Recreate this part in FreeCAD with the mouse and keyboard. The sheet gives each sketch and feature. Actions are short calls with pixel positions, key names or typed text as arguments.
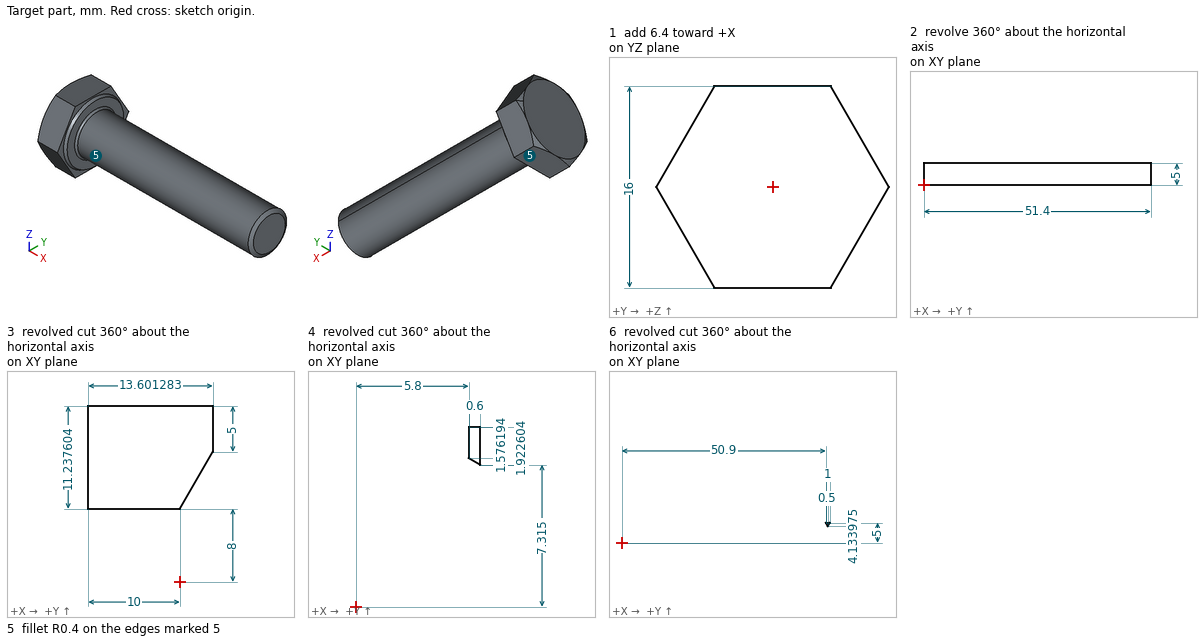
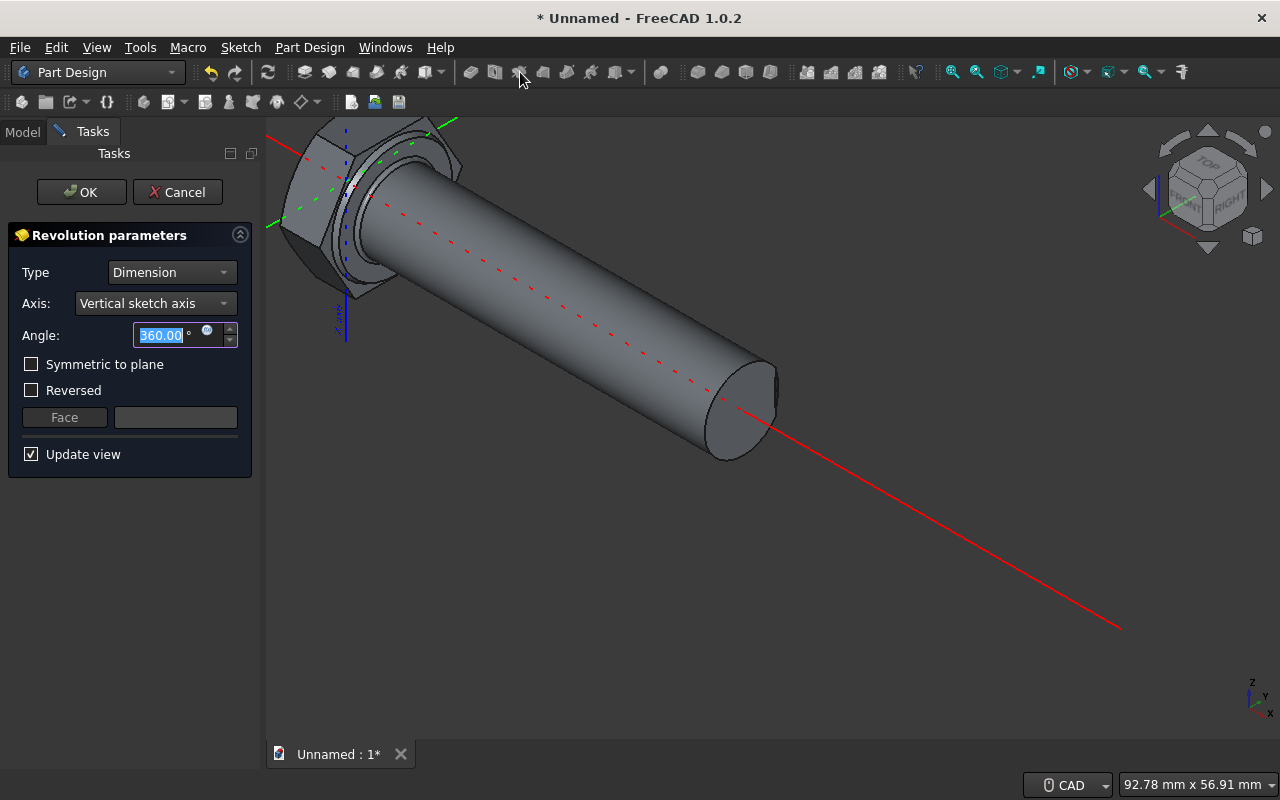
click(156, 304)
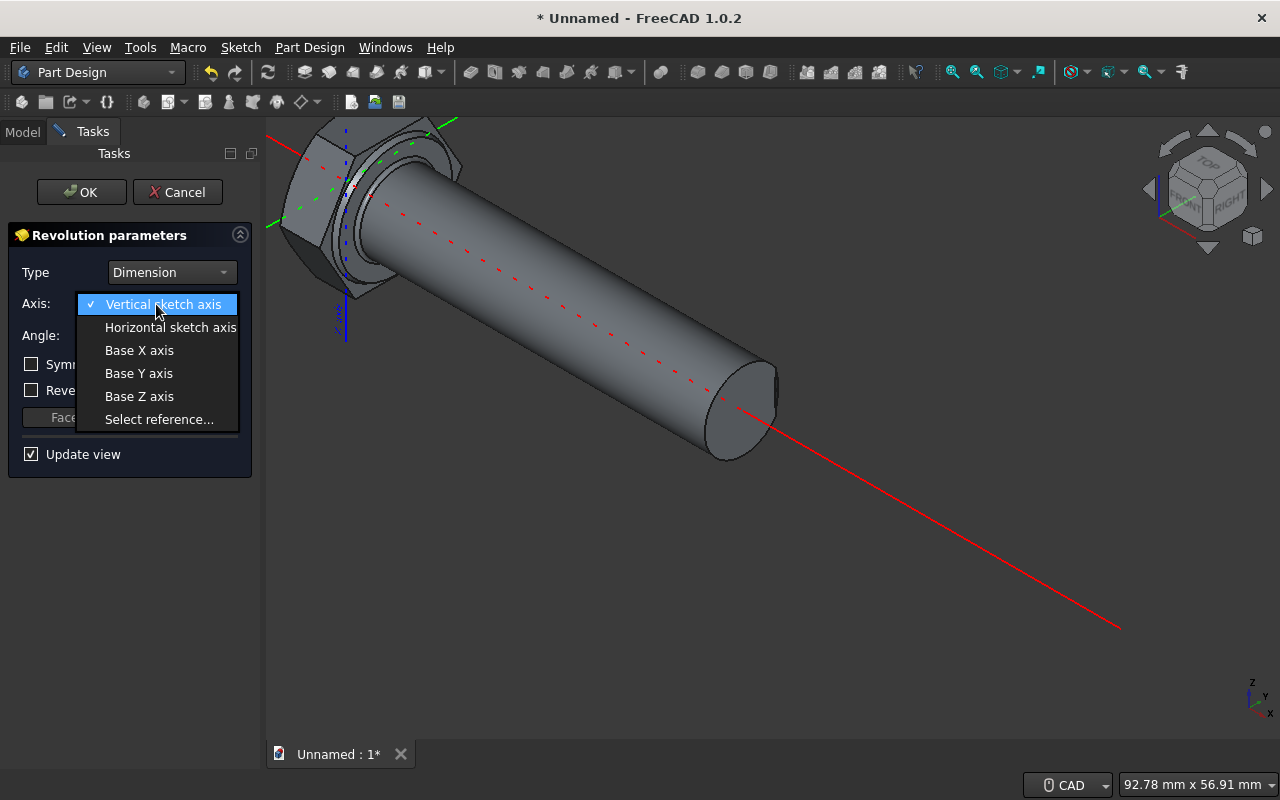
click(156, 328)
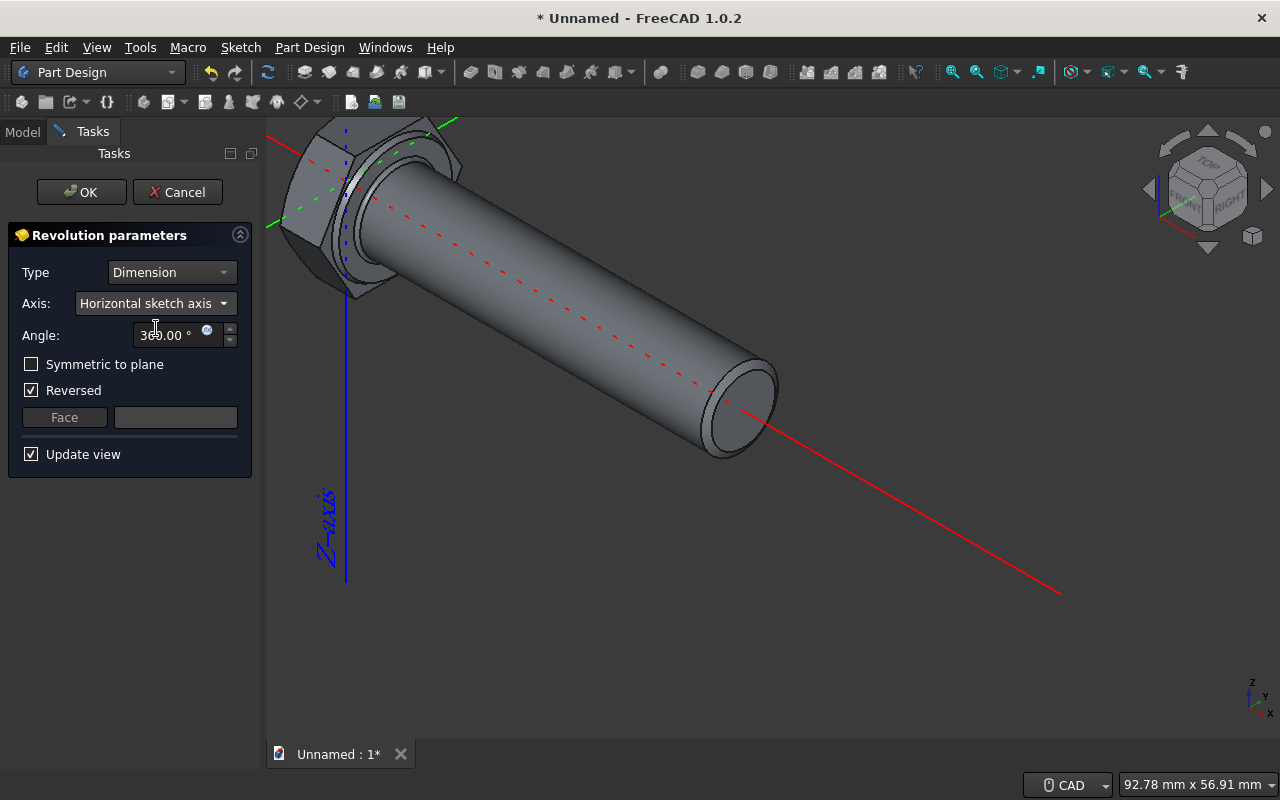
click(82, 192)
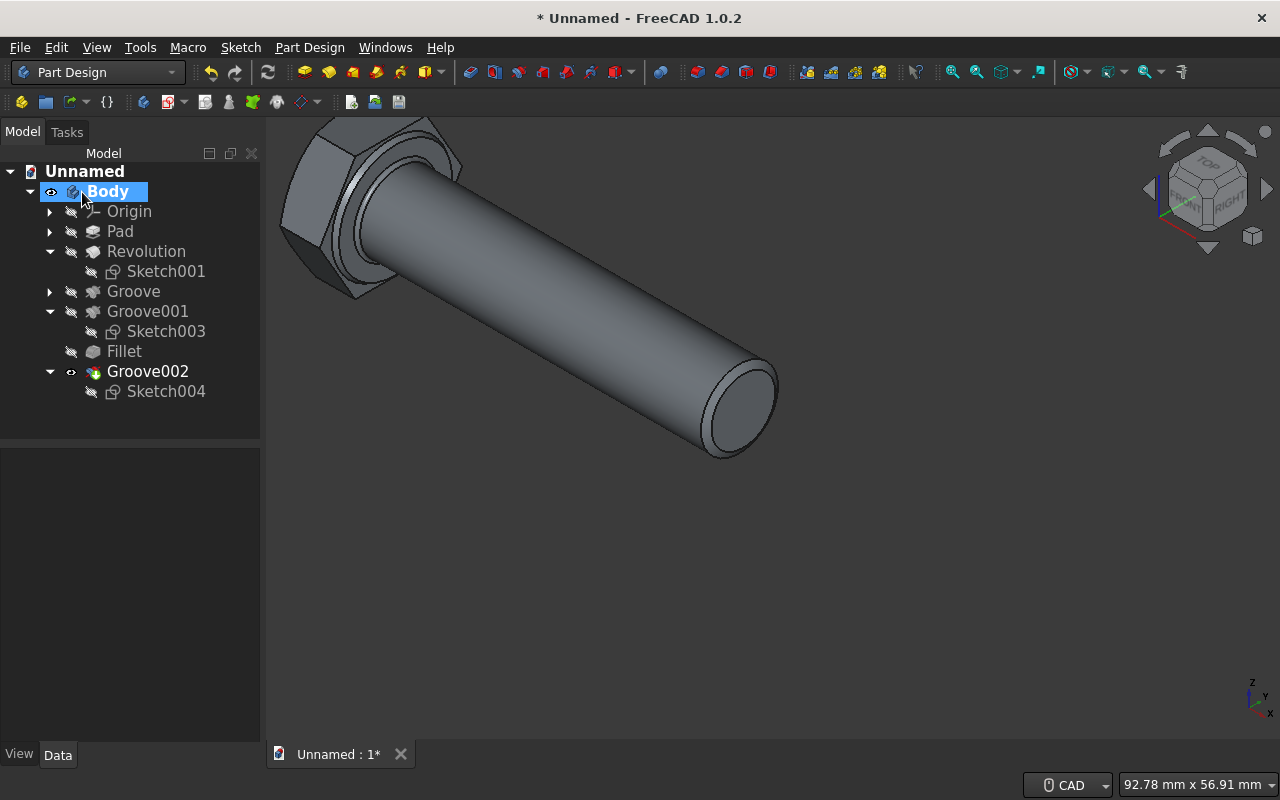
click(954, 72)